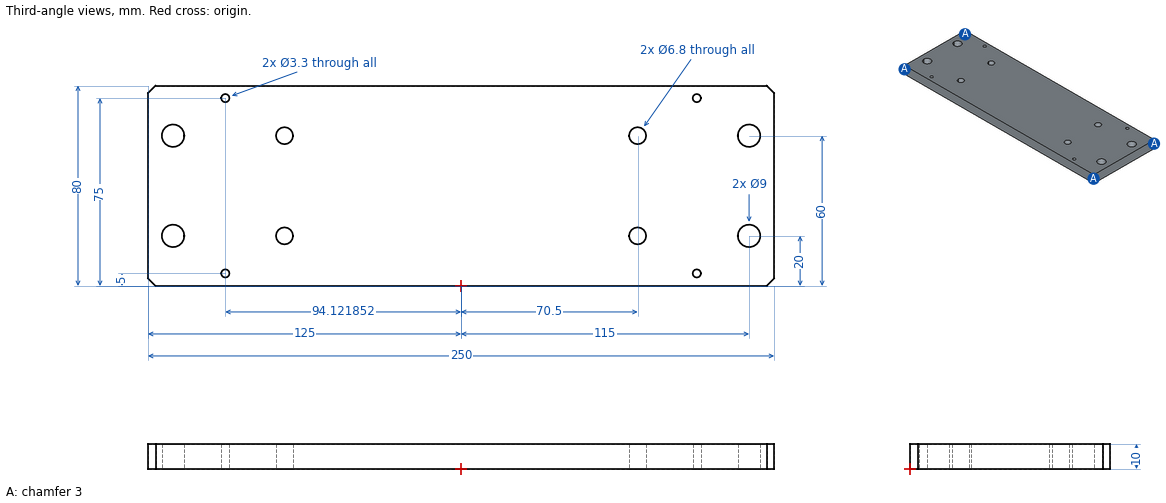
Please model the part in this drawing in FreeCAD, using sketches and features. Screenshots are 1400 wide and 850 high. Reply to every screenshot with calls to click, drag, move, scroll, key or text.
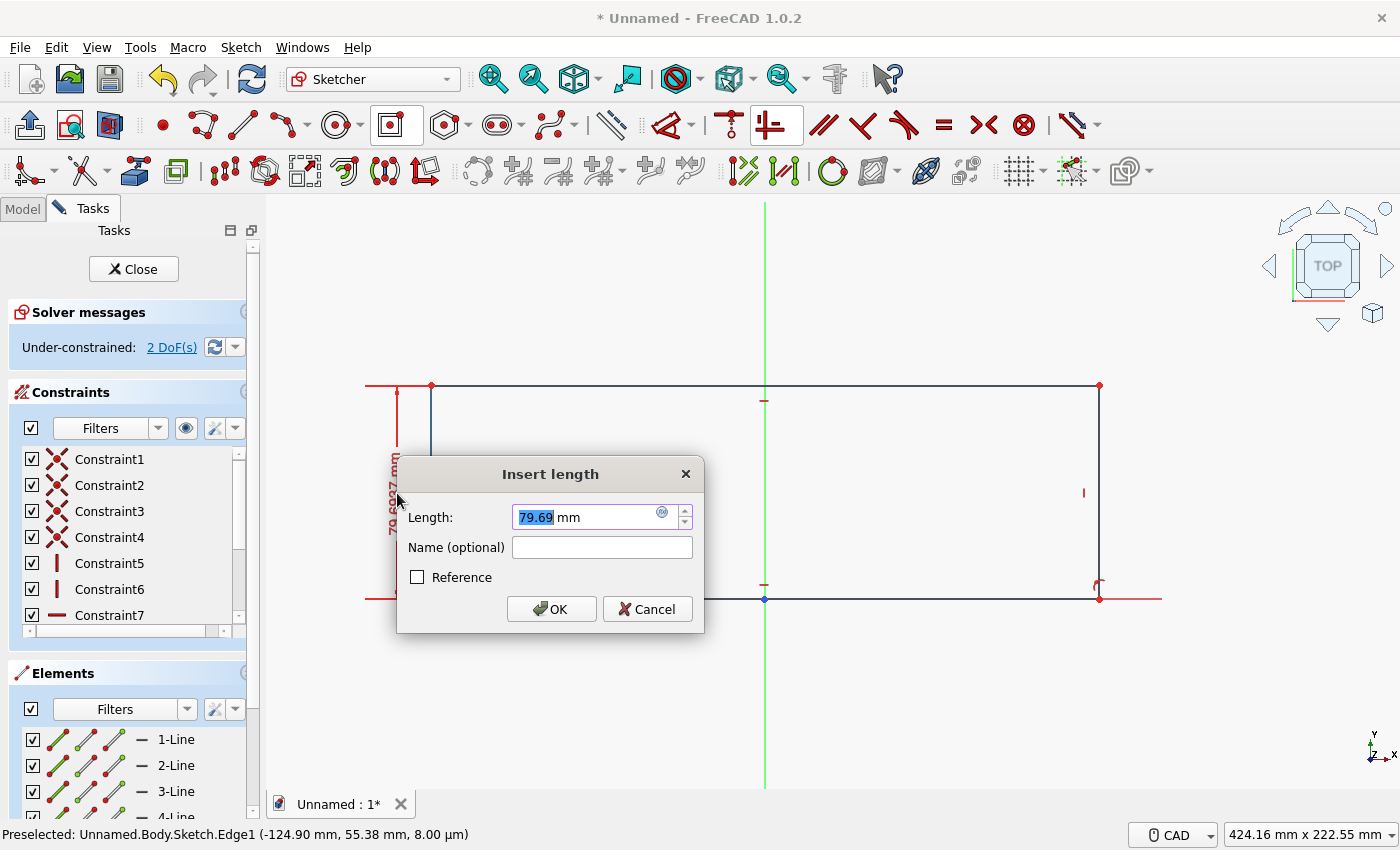
text(80)
key(Return)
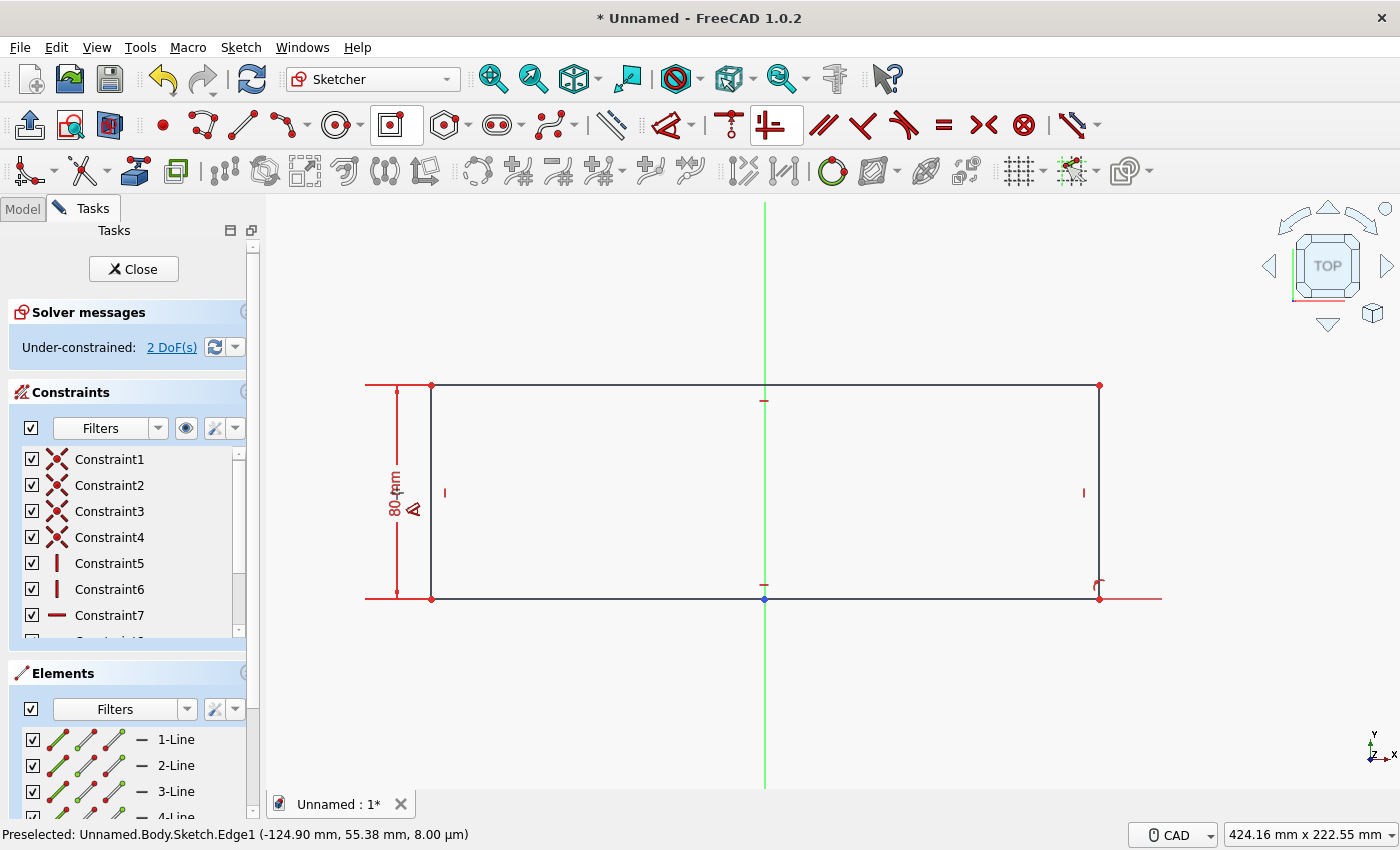
click(631, 599)
click(611, 633)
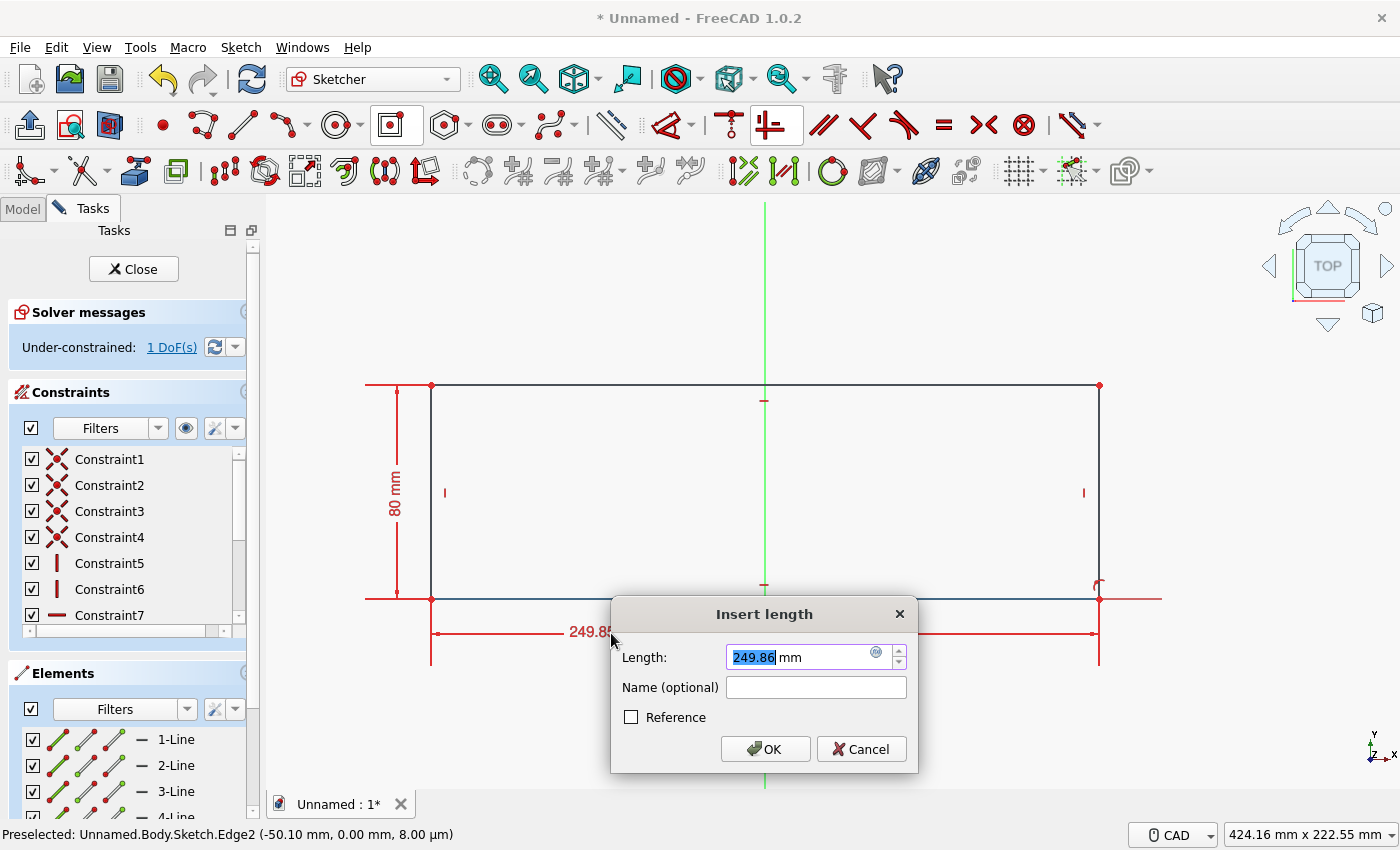
text(250)
key(Return)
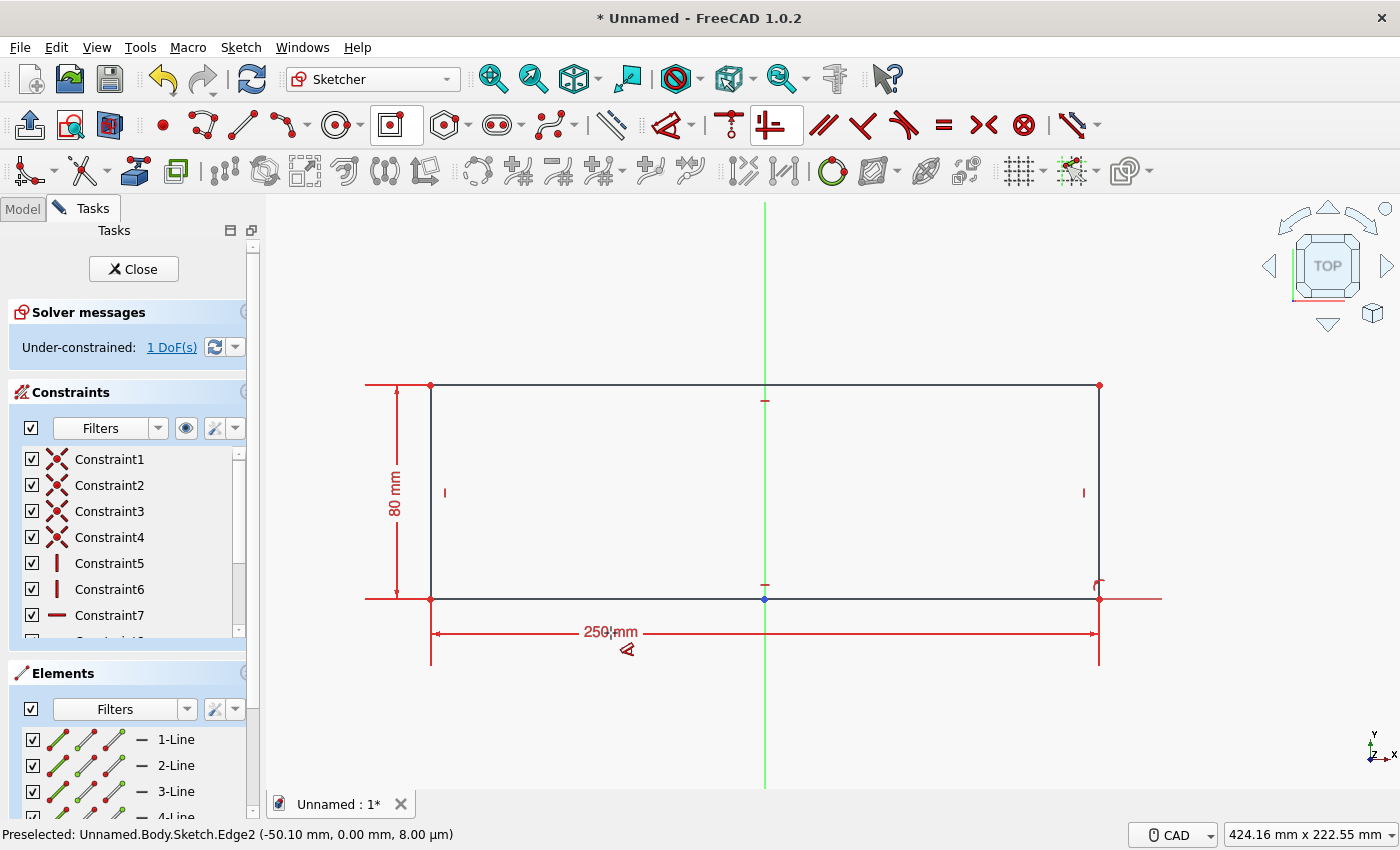
click(431, 385)
click(521, 633)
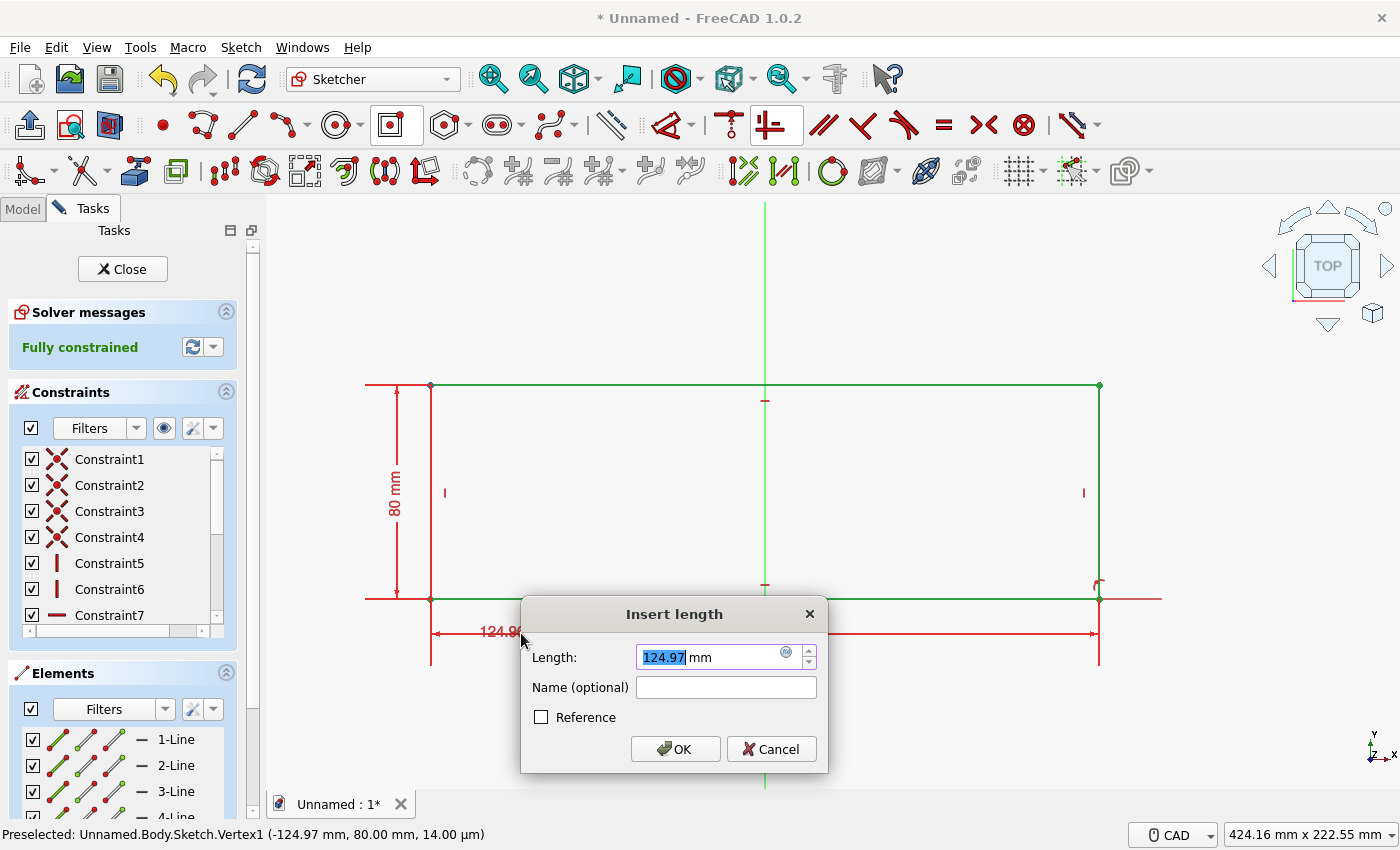
text(125)
key(Return)
key(Escape)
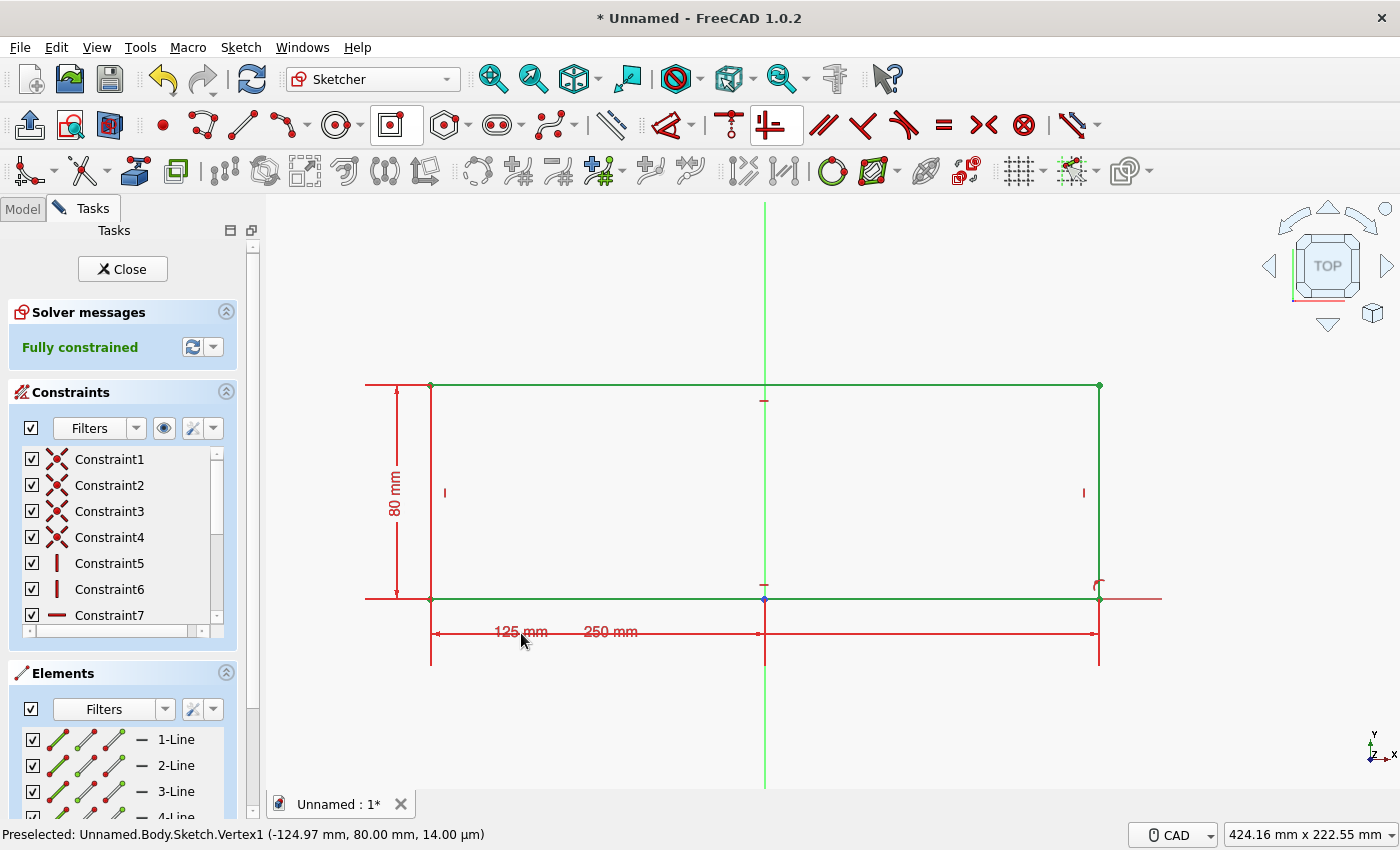
click(123, 269)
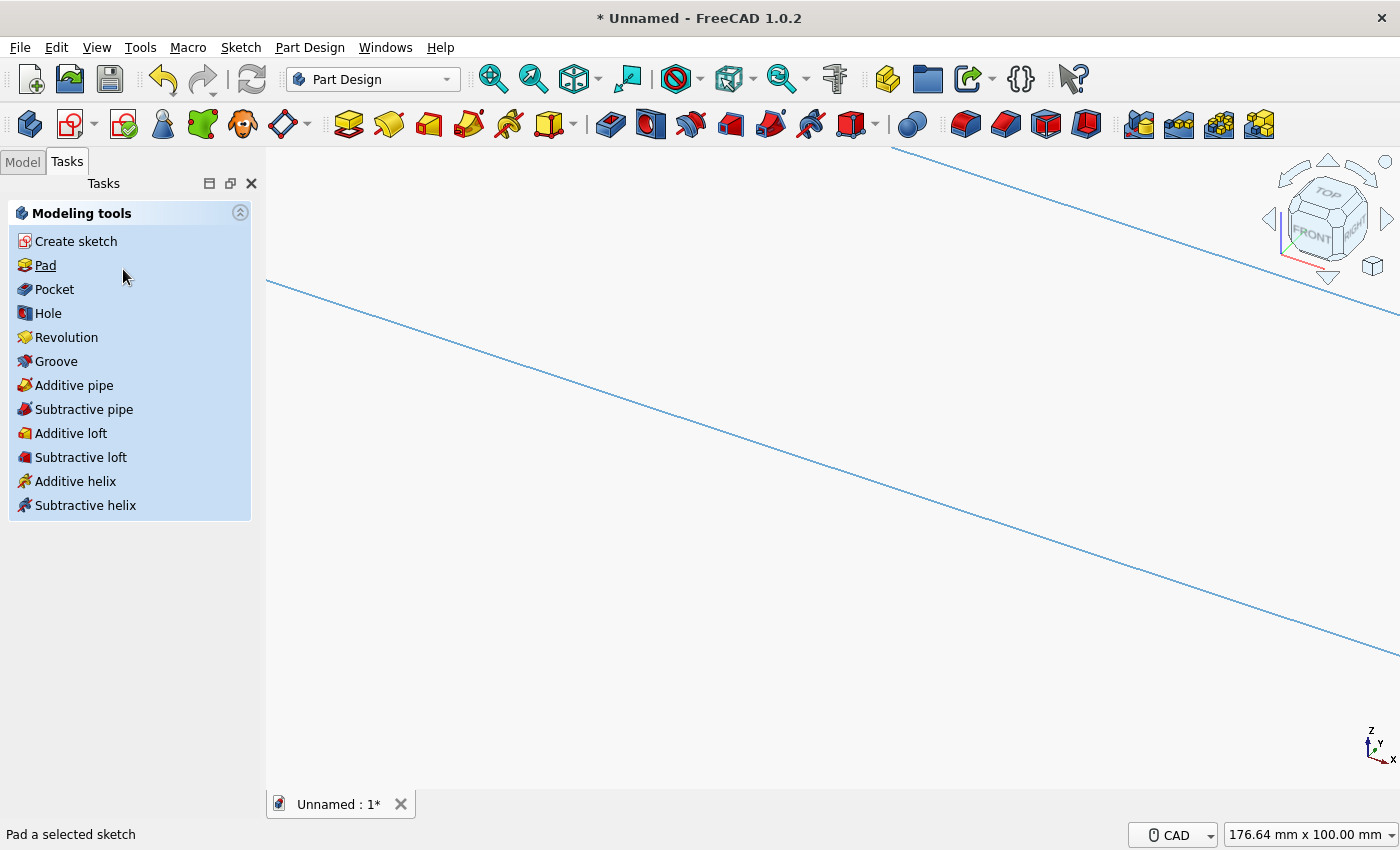
click(350, 124)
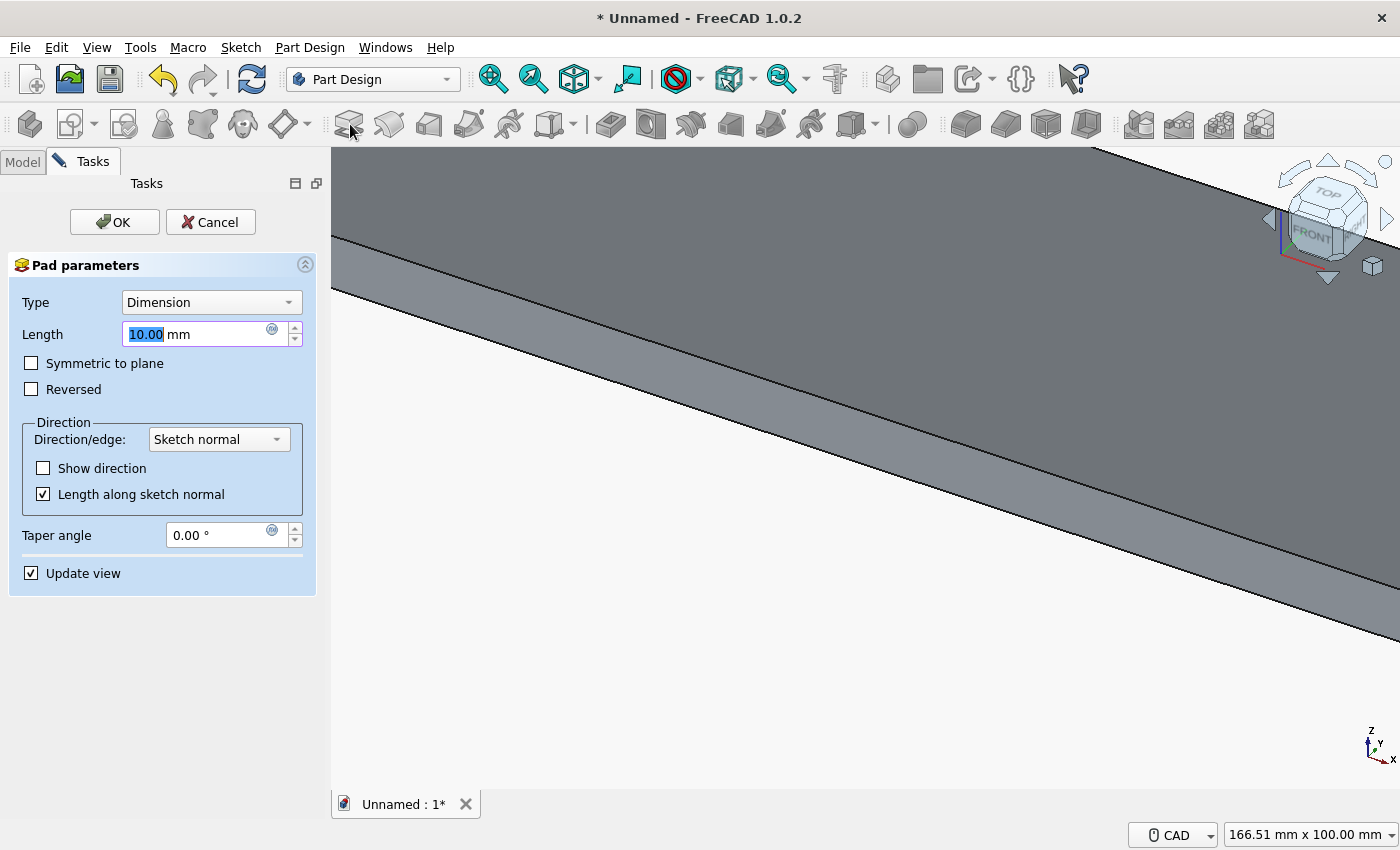
text(10)
key(Tab)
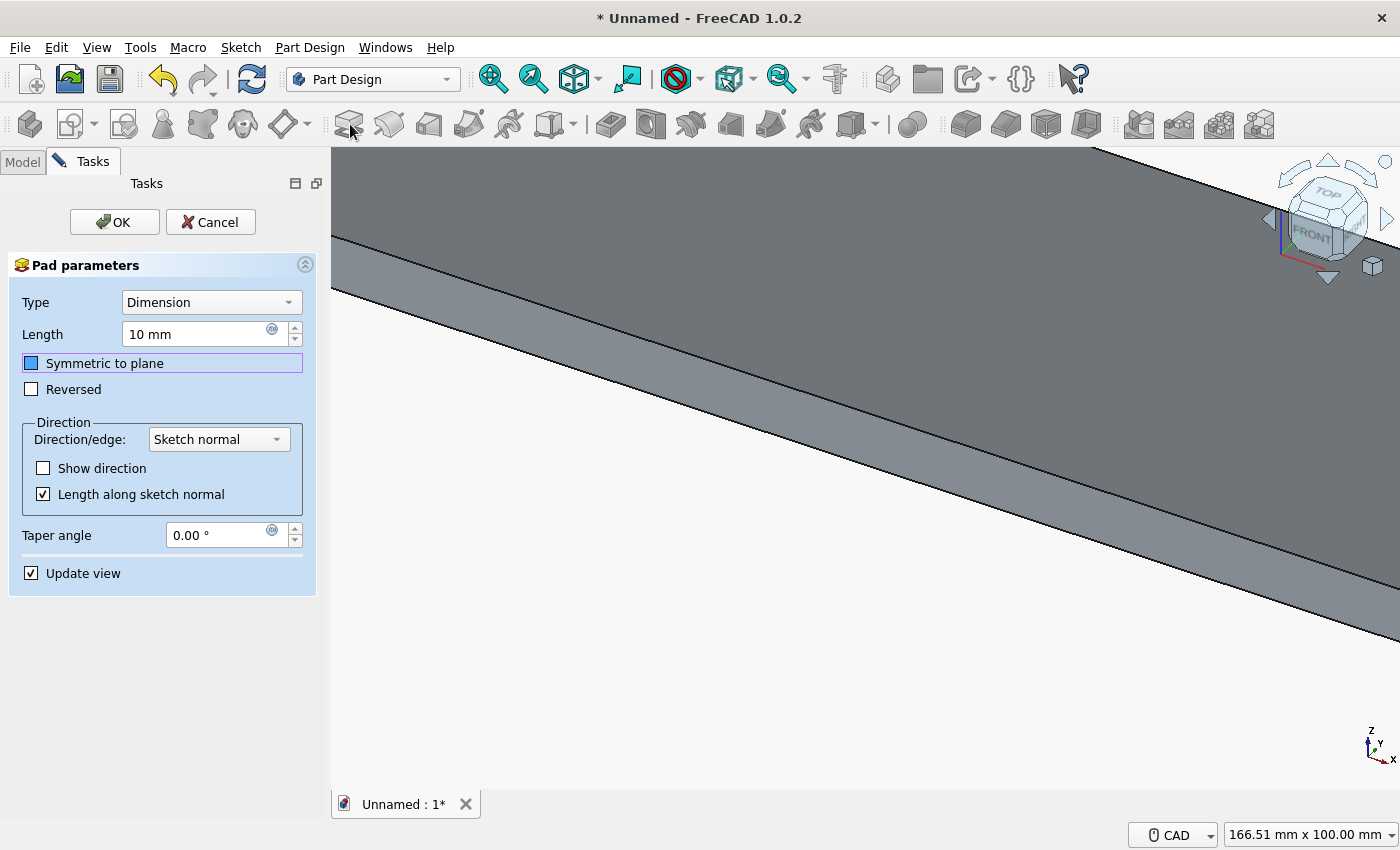
click(115, 222)